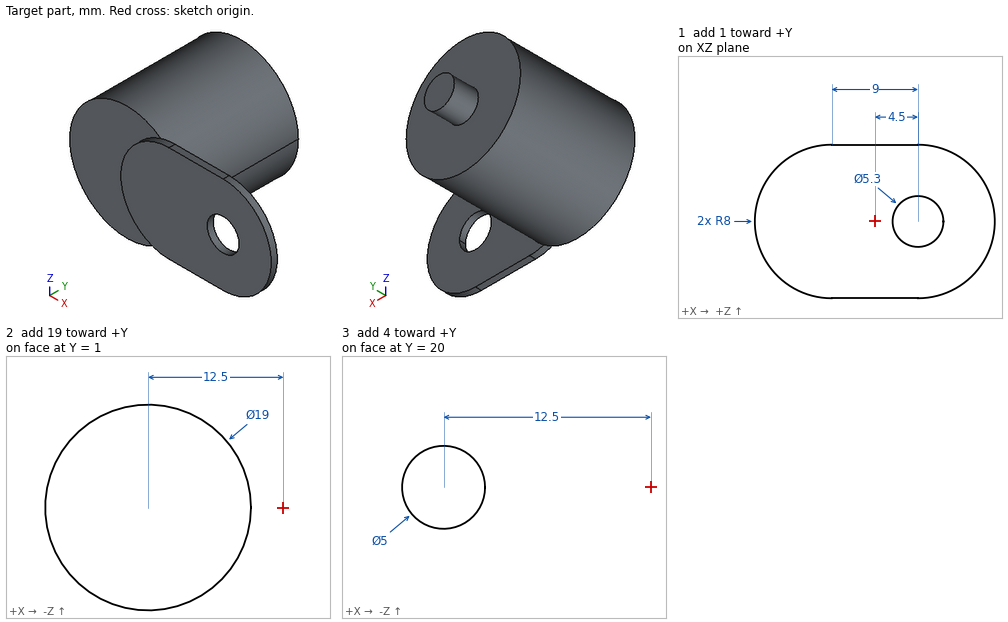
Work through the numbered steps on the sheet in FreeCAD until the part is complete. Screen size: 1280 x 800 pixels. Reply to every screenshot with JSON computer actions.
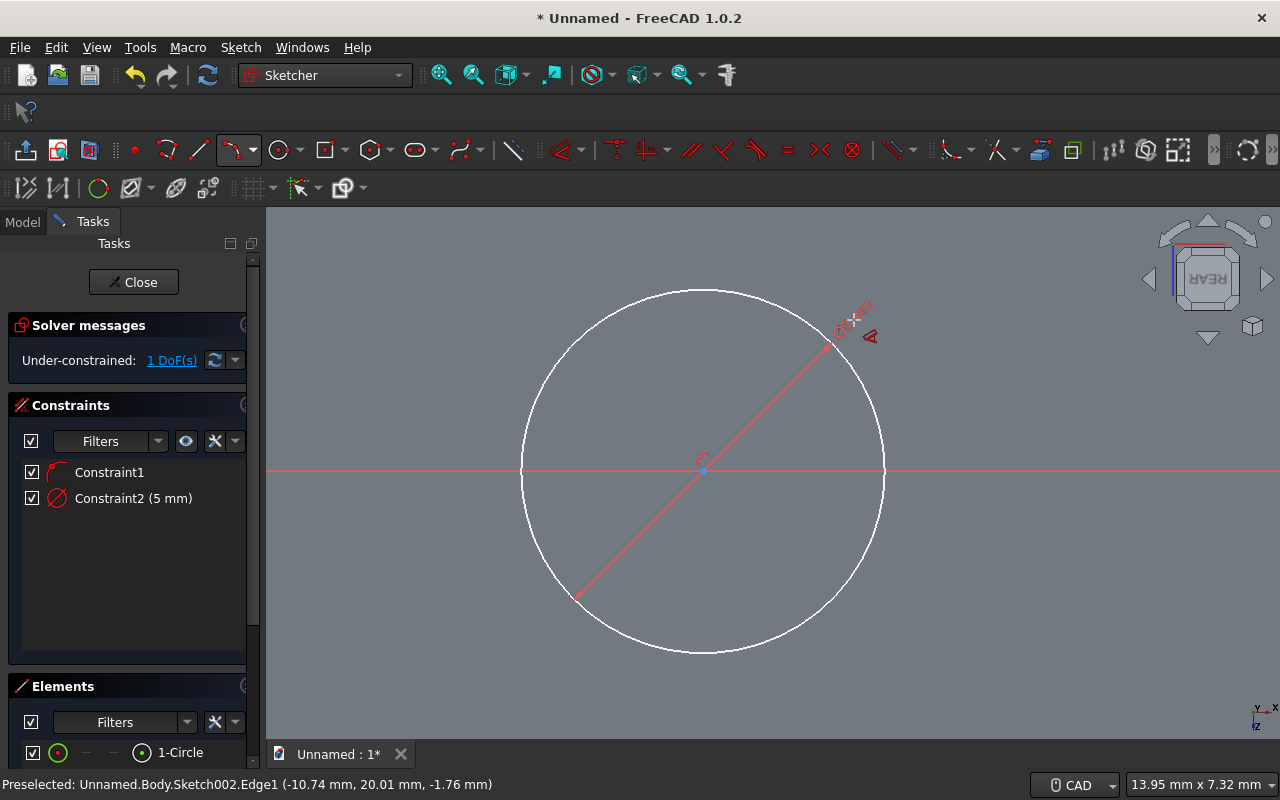
{"action": "left_click", "coordinate": [703, 471]}
{"action": "left_click", "coordinate": [909, 505]}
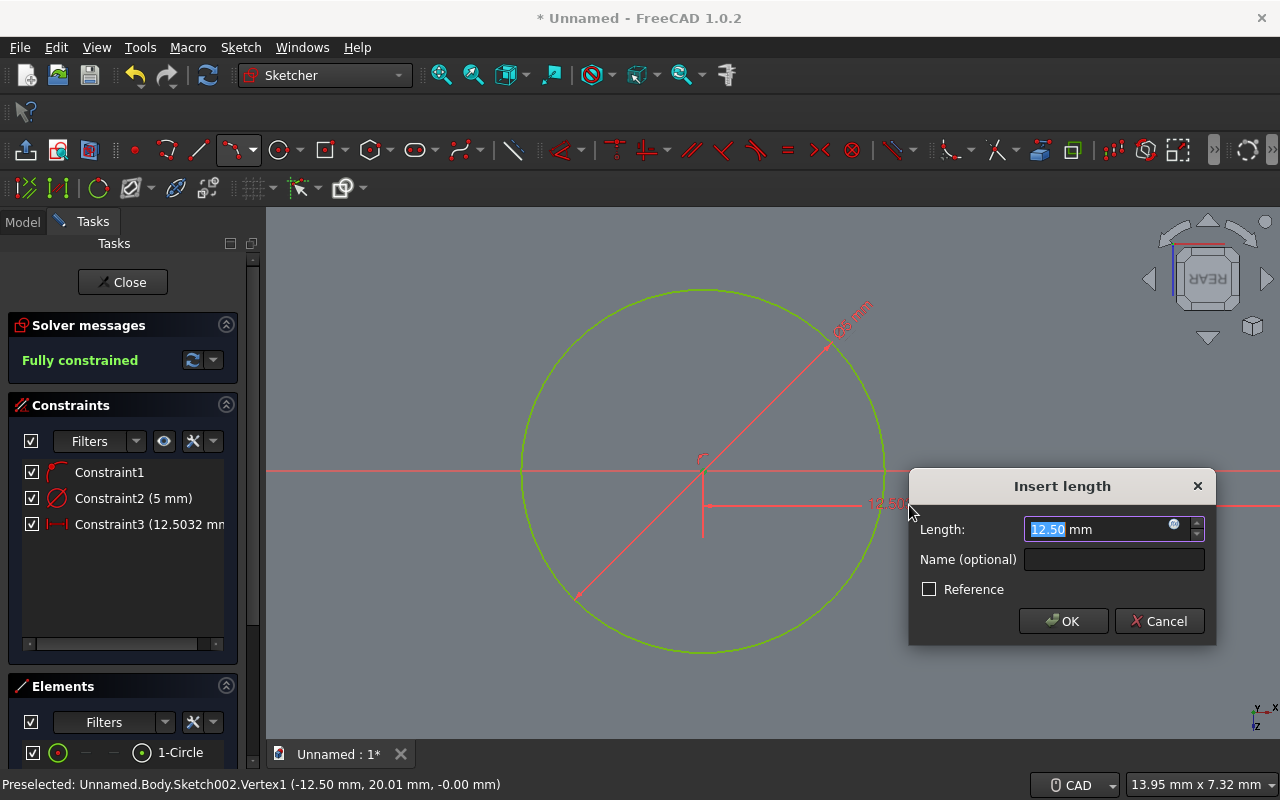
{"action": "type", "text": "12.5"}
{"action": "key", "text": "Return"}
{"action": "key", "text": "Escape"}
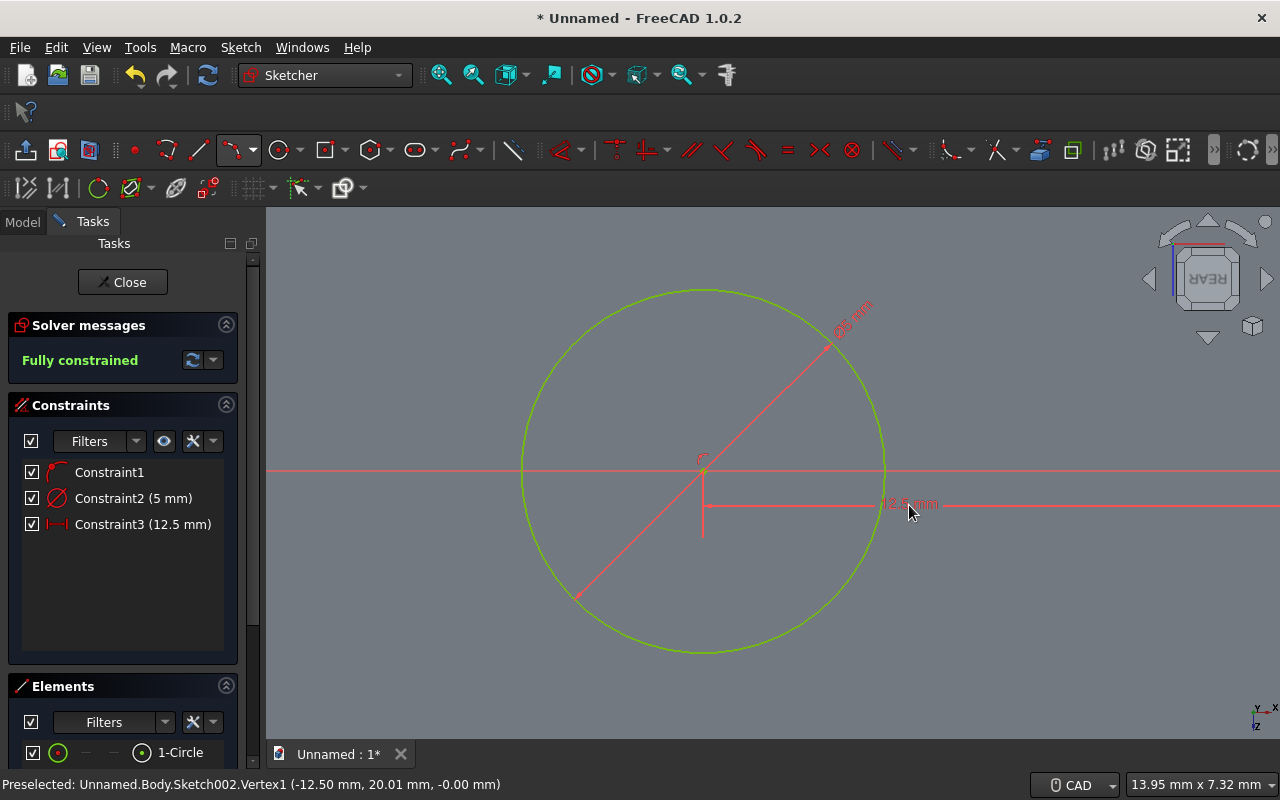
{"action": "left_click", "coordinate": [123, 282]}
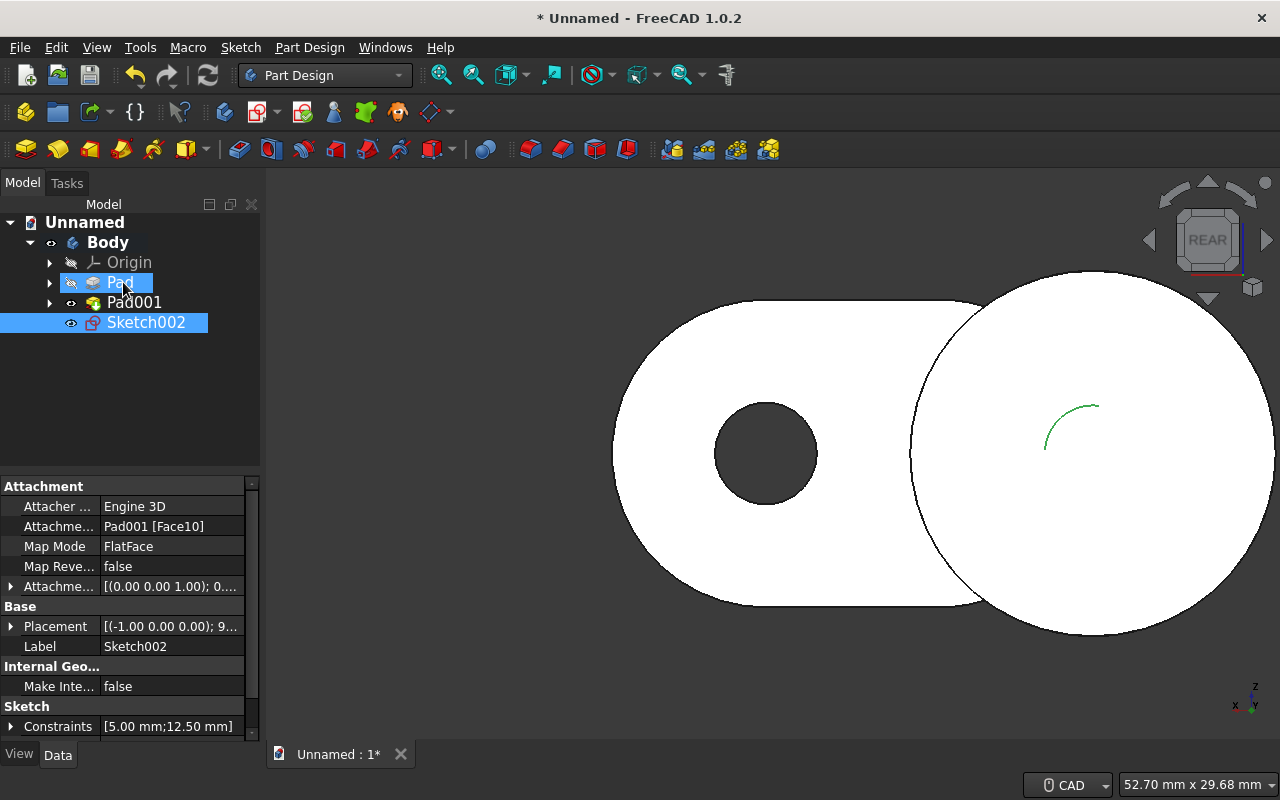
{"action": "left_click", "coordinate": [26, 150]}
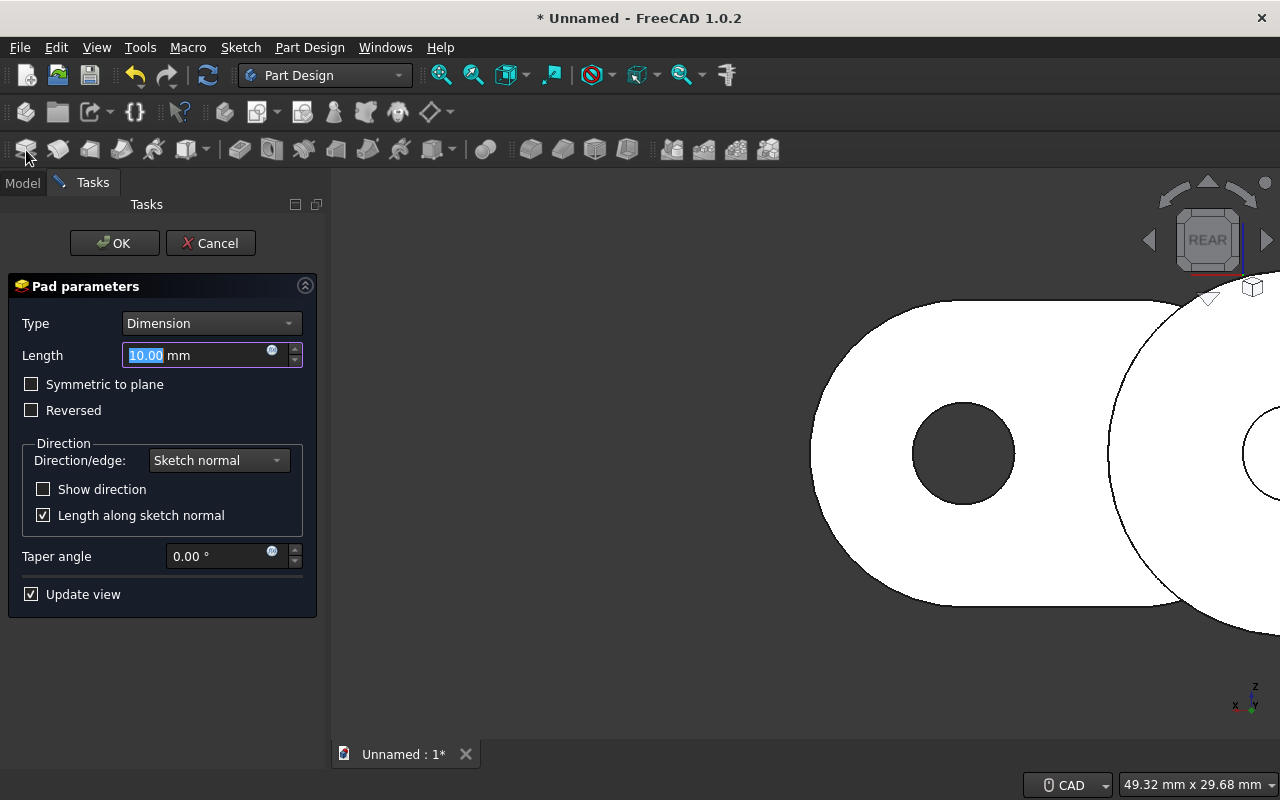
{"action": "type", "text": "4"}
{"action": "key", "text": "Tab"}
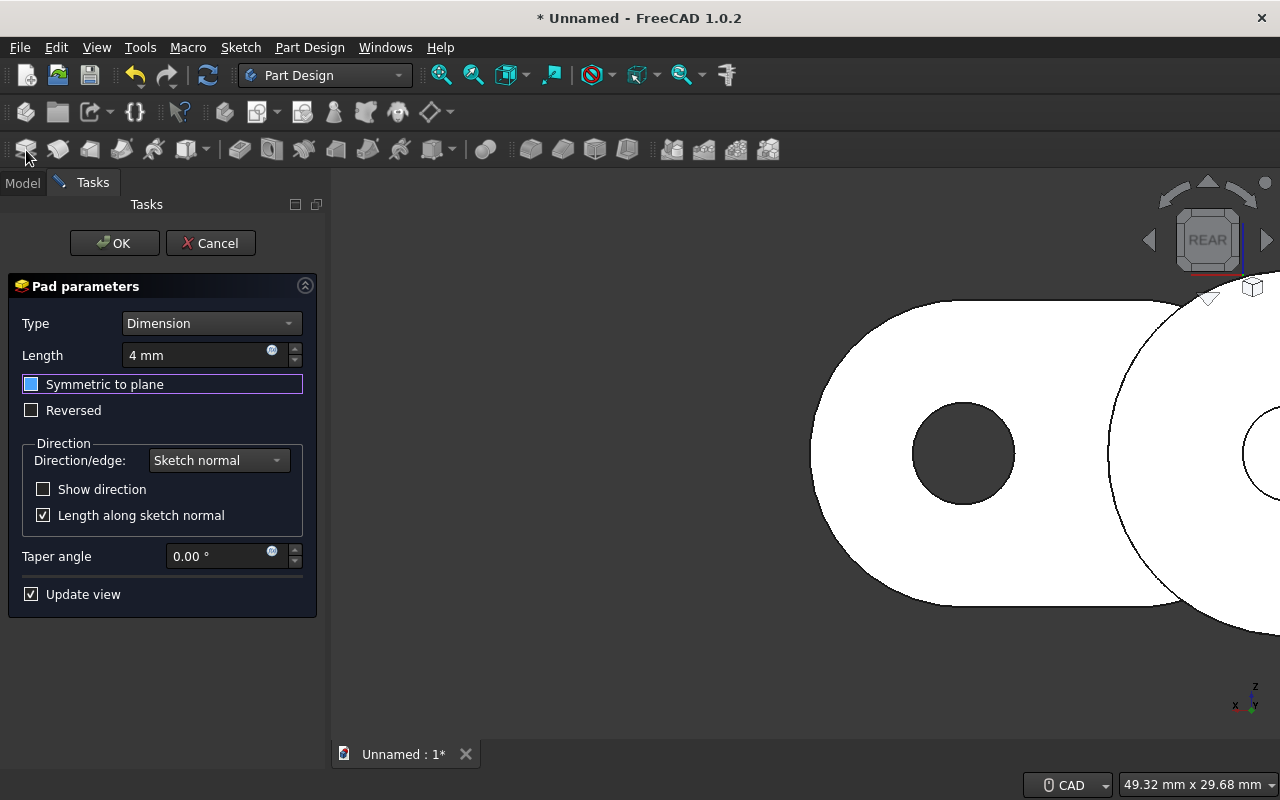
{"action": "left_click", "coordinate": [115, 243]}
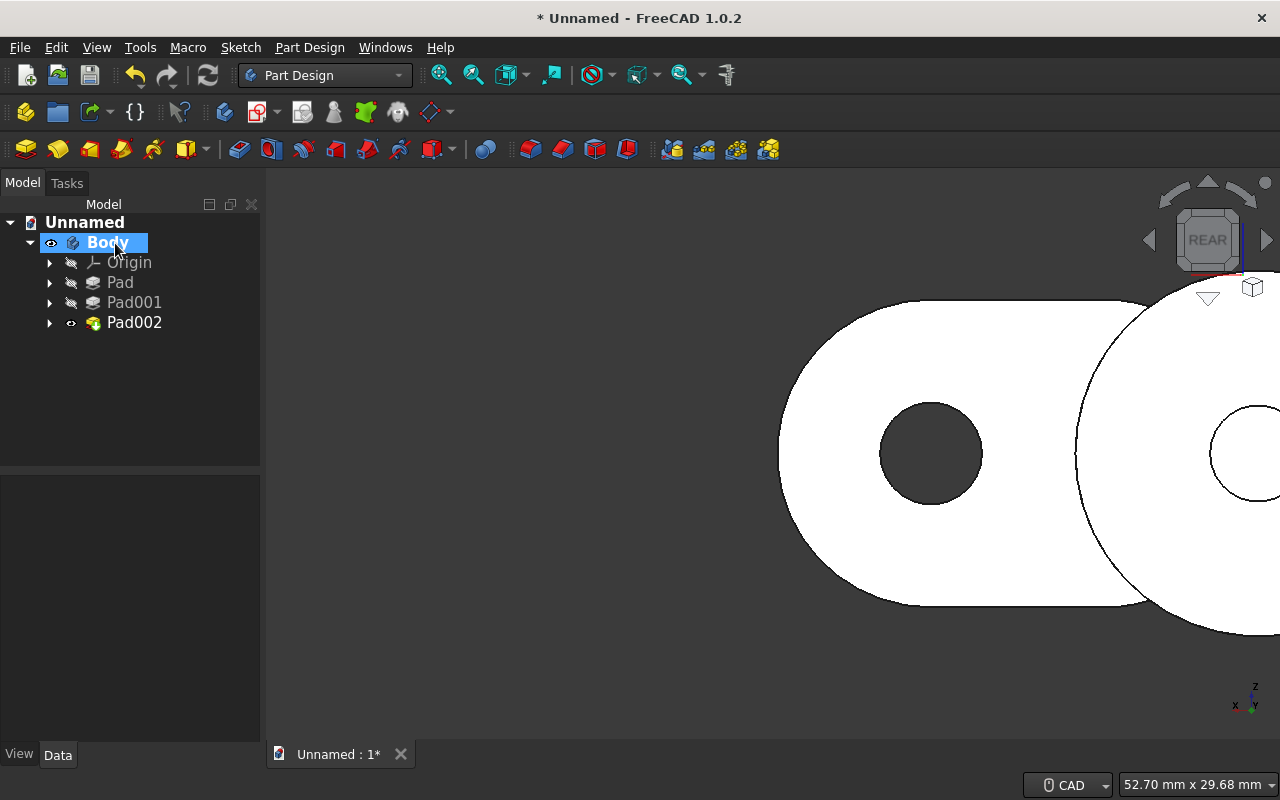
{"action": "key", "text": "0"}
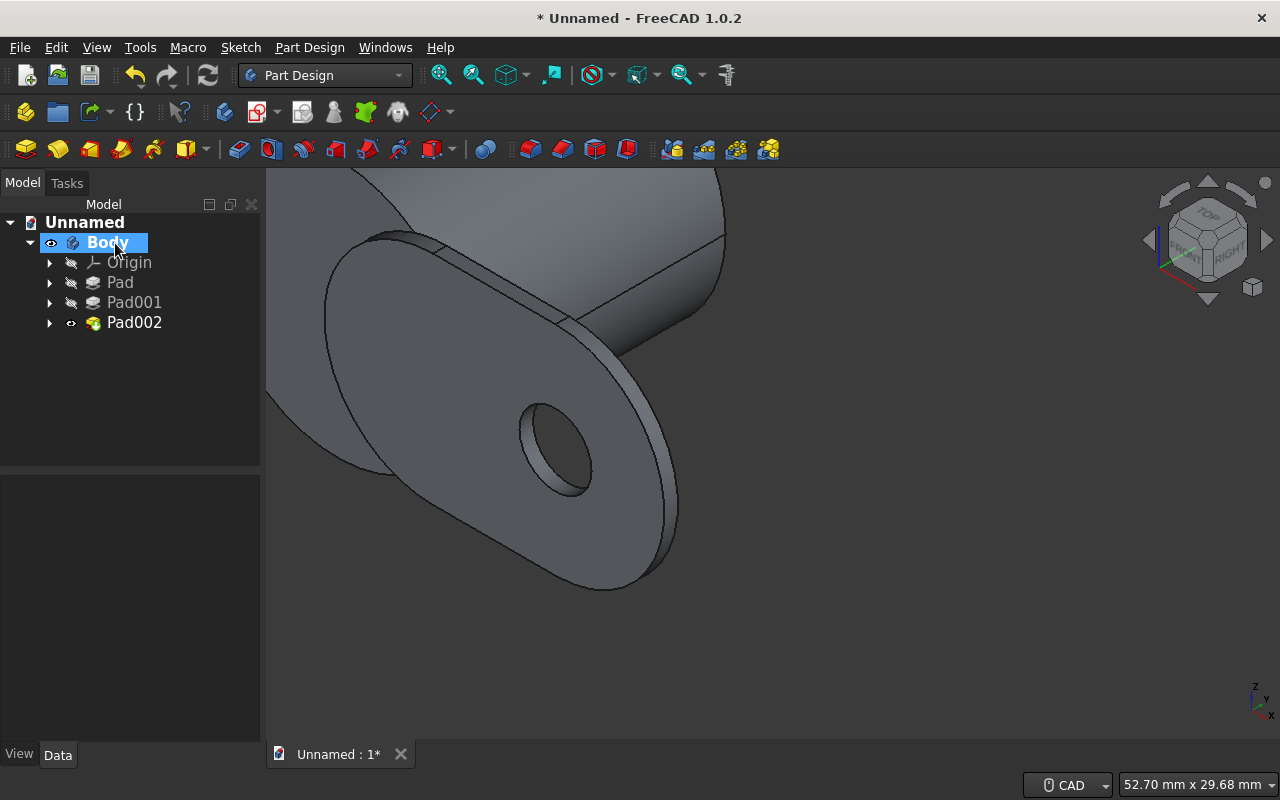
{"action": "left_click", "coordinate": [442, 76]}